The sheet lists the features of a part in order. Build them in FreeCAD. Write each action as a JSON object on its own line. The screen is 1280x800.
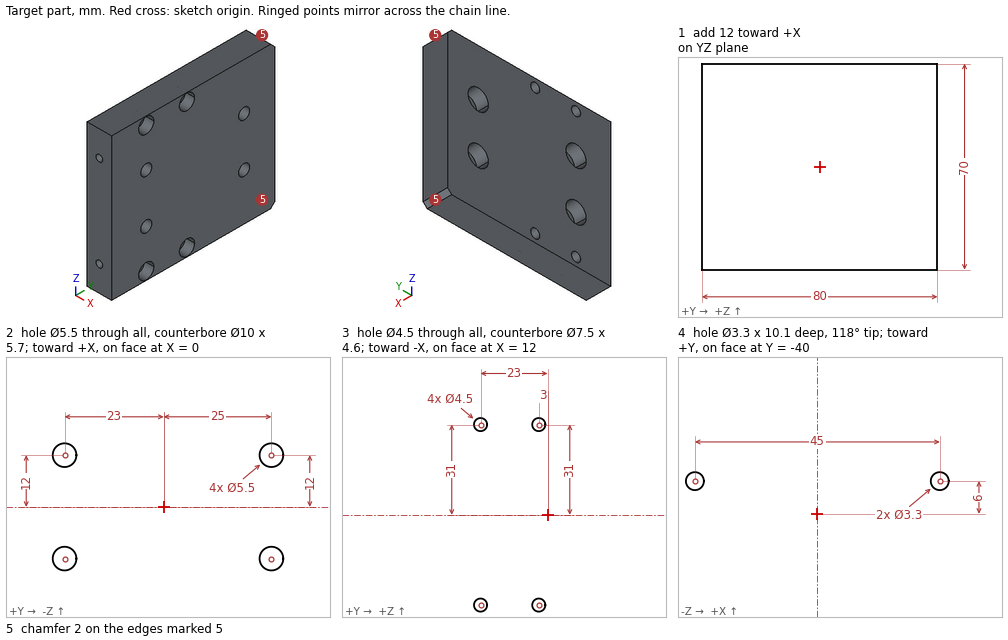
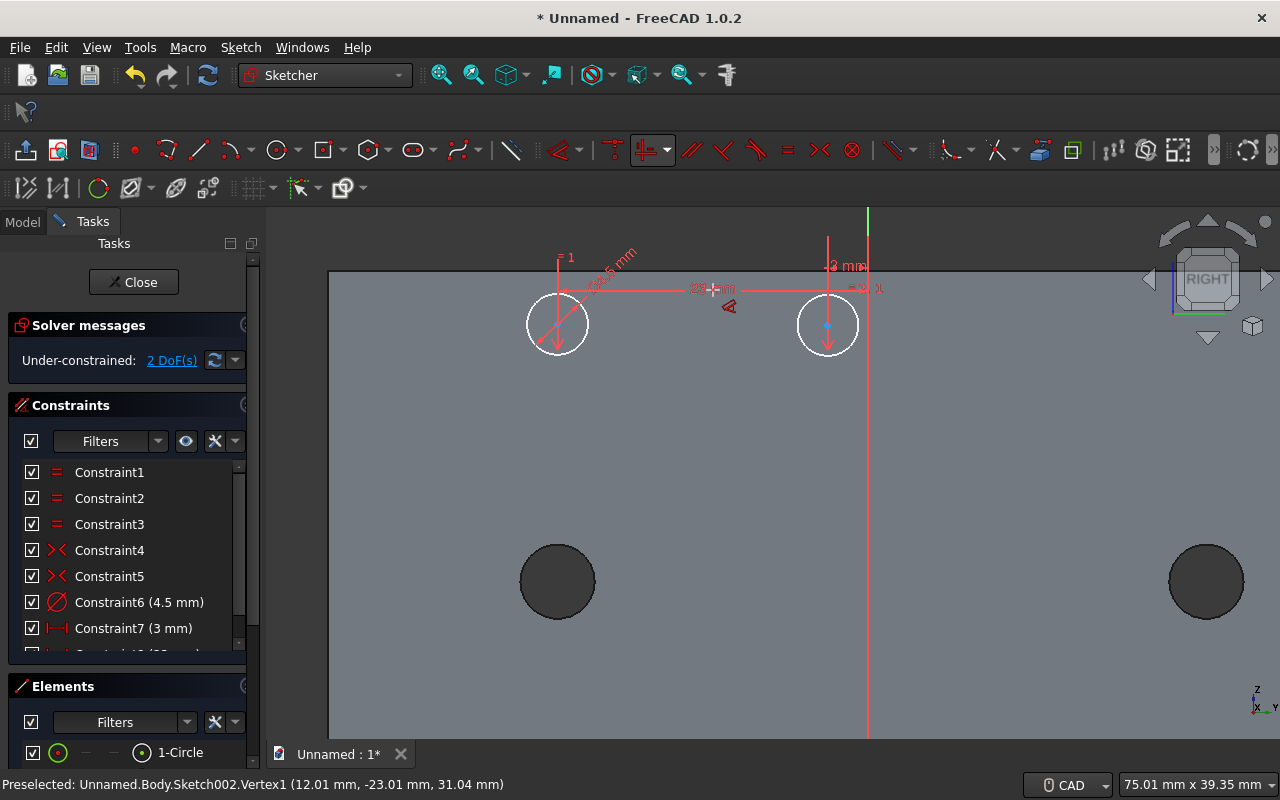
{"action": "left_click", "coordinate": [558, 324]}
{"action": "left_click", "coordinate": [902, 518]}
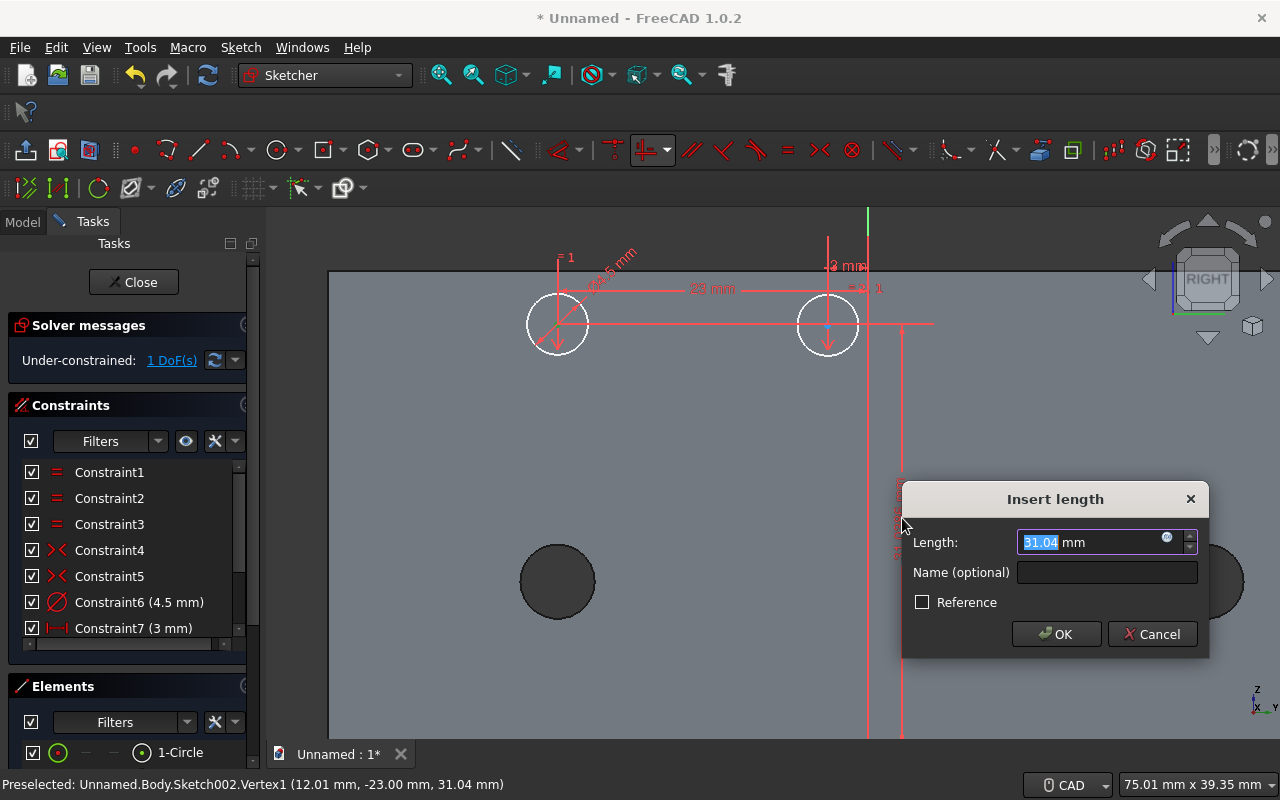
{"action": "type", "text": "31"}
{"action": "key", "text": "Return"}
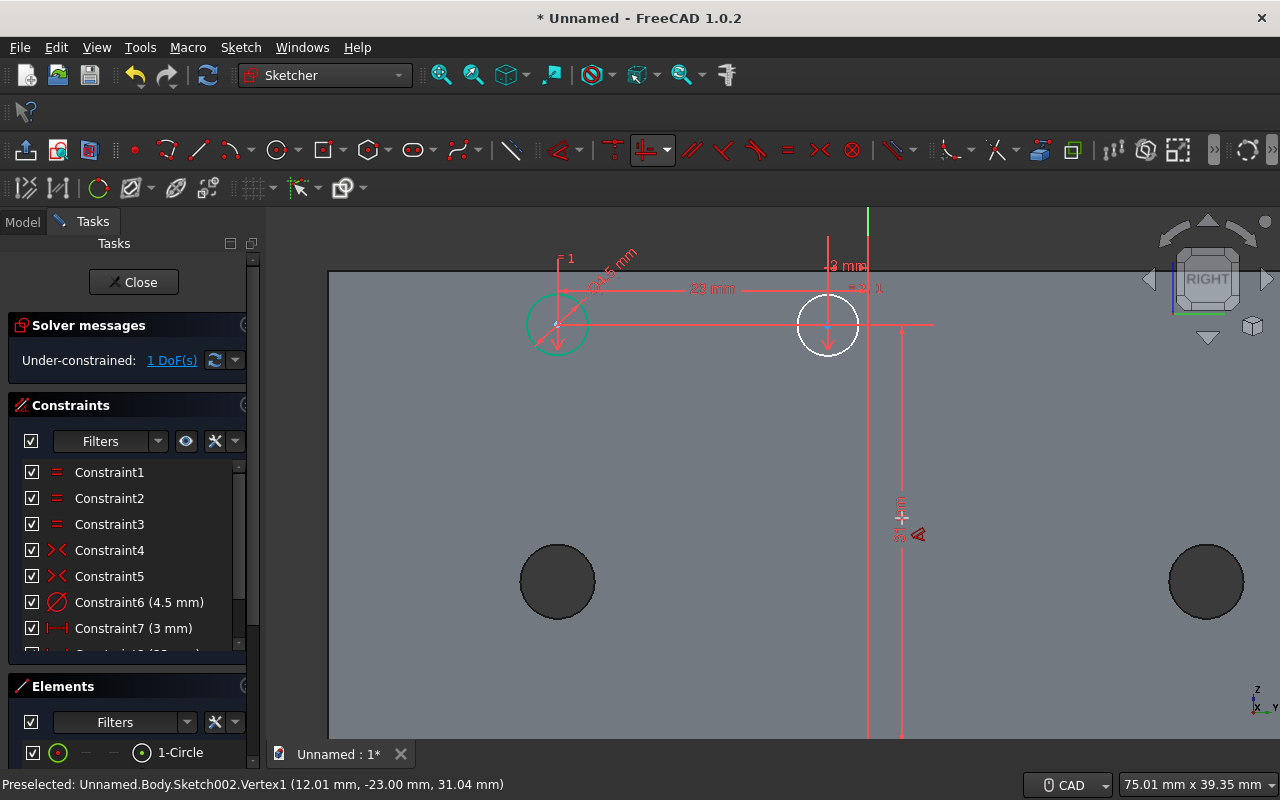
{"action": "left_click", "coordinate": [828, 325]}
{"action": "left_click", "coordinate": [902, 430]}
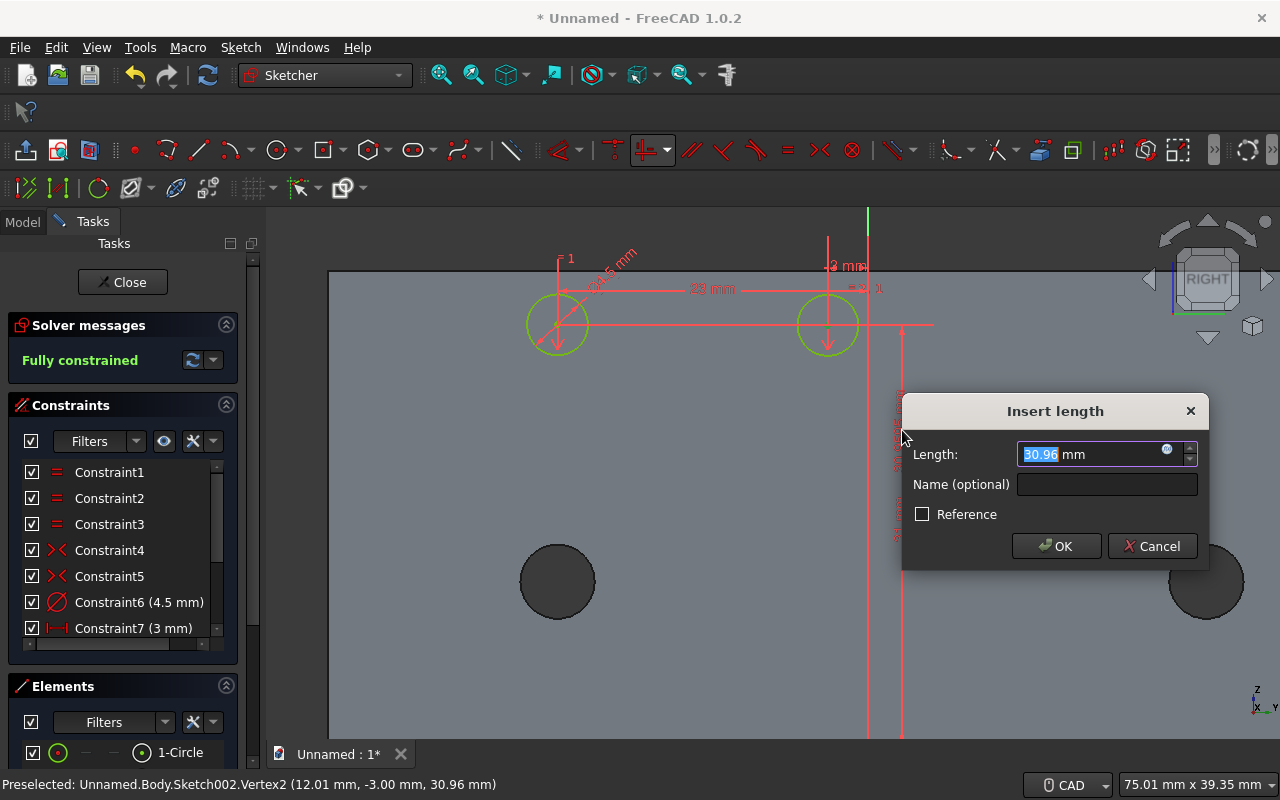
{"action": "type", "text": "31"}
{"action": "key", "text": "Return"}
{"action": "key", "text": "Escape"}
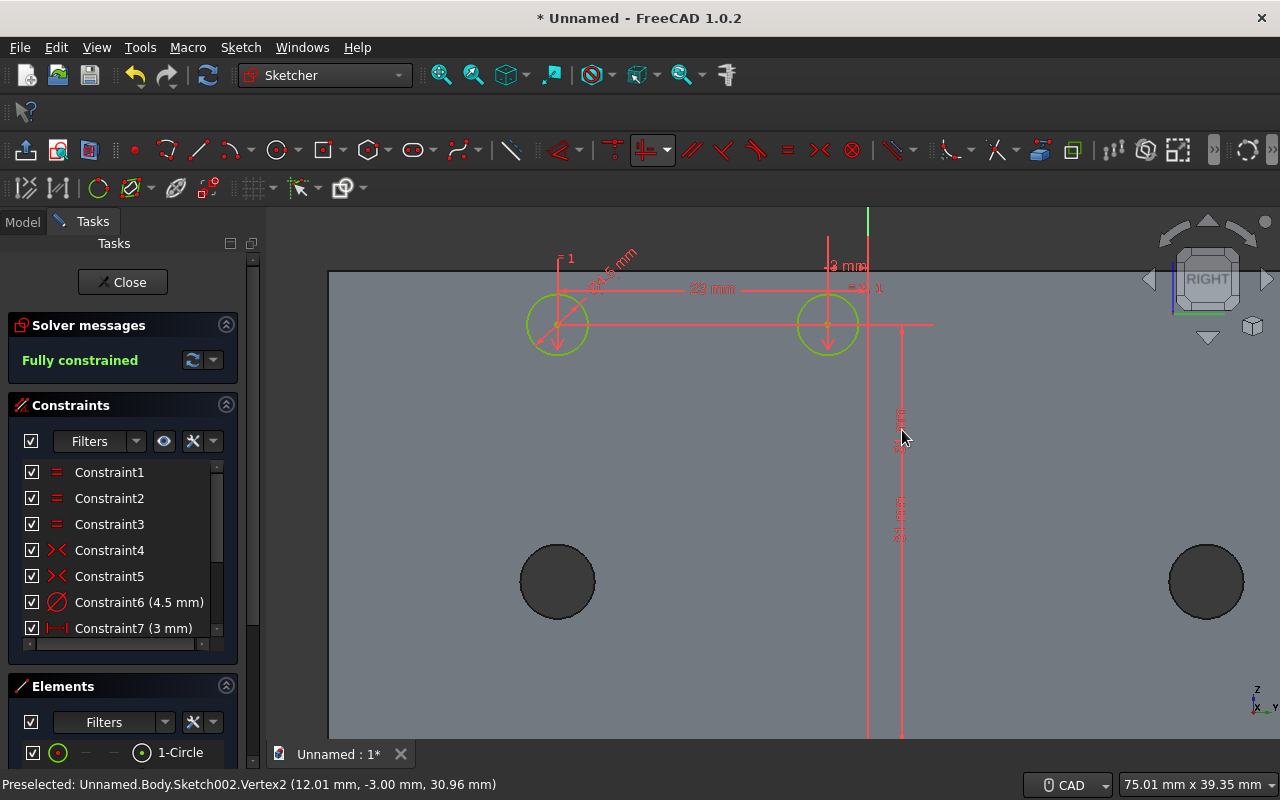
{"action": "left_click", "coordinate": [123, 282]}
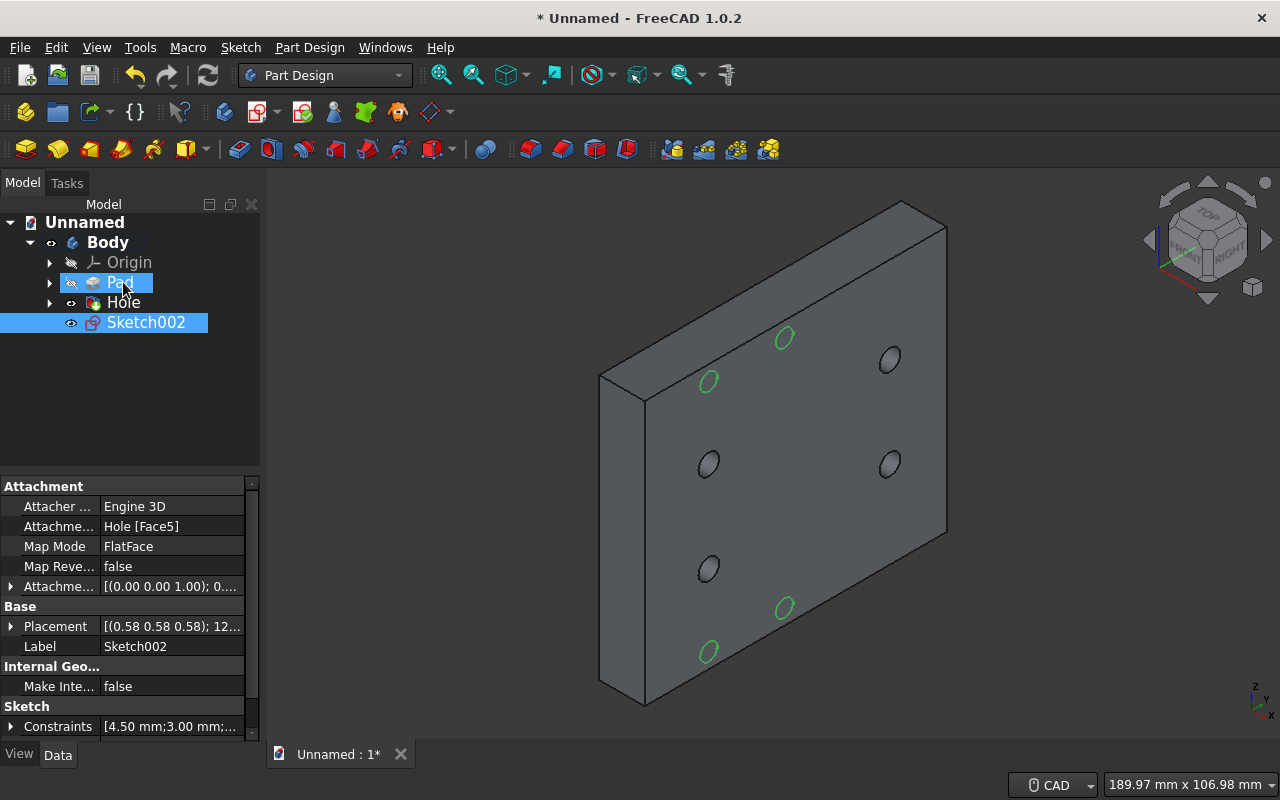
{"action": "left_click", "coordinate": [272, 150]}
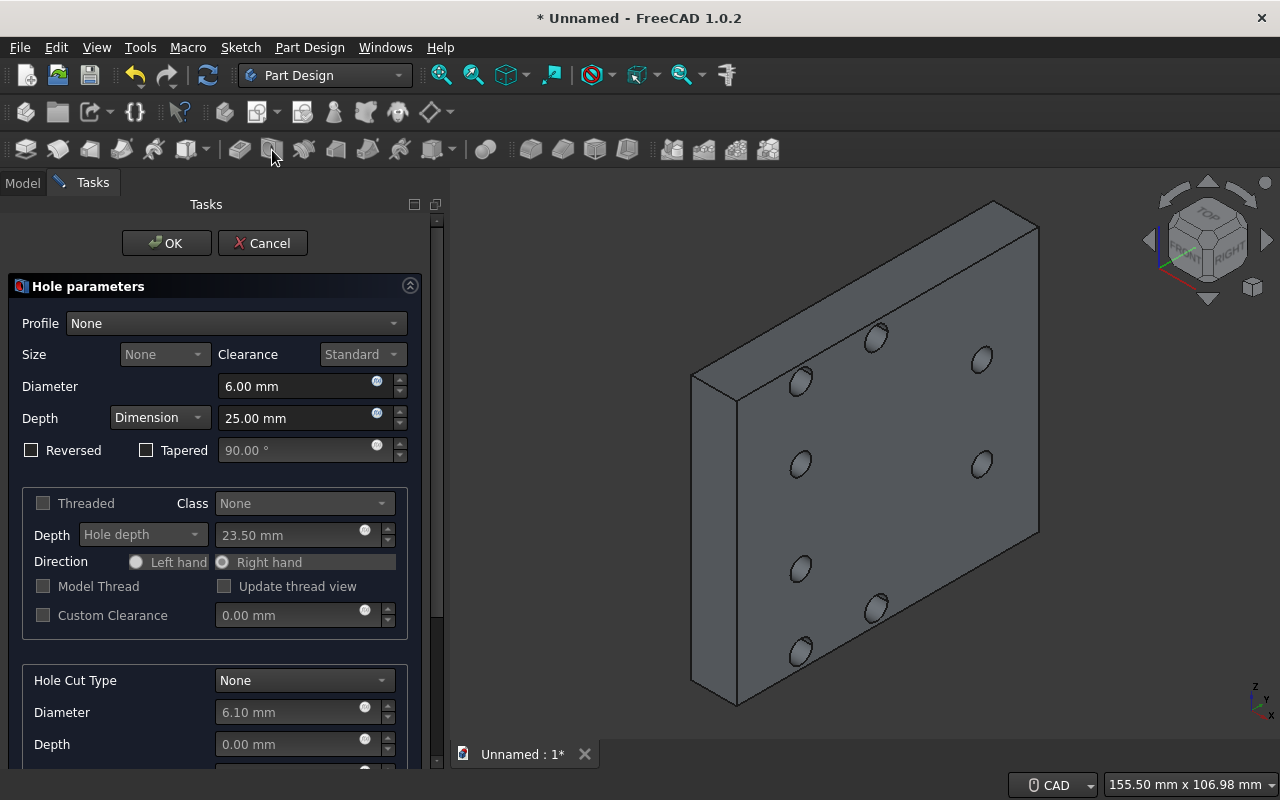
{"action": "triple_click", "coordinate": [305, 386]}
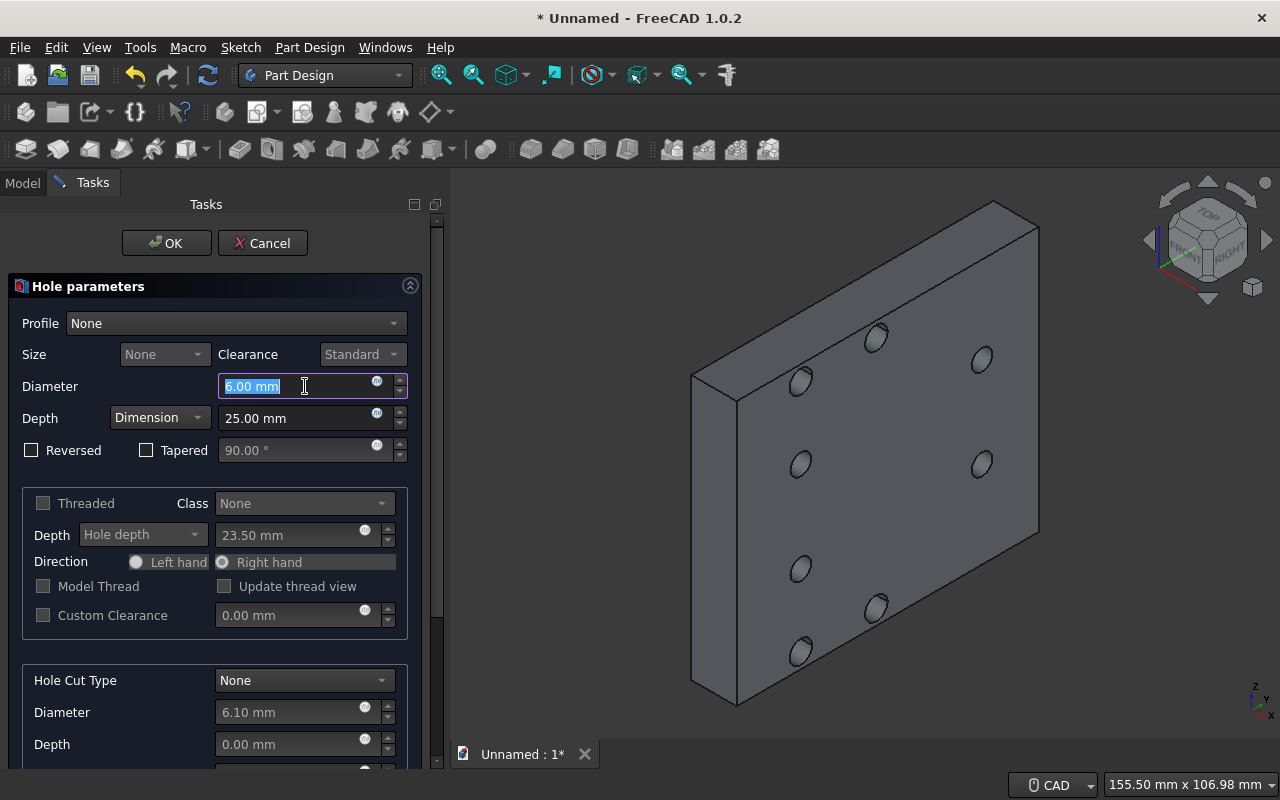
{"action": "type", "text": "4.5"}
{"action": "key", "text": "Tab"}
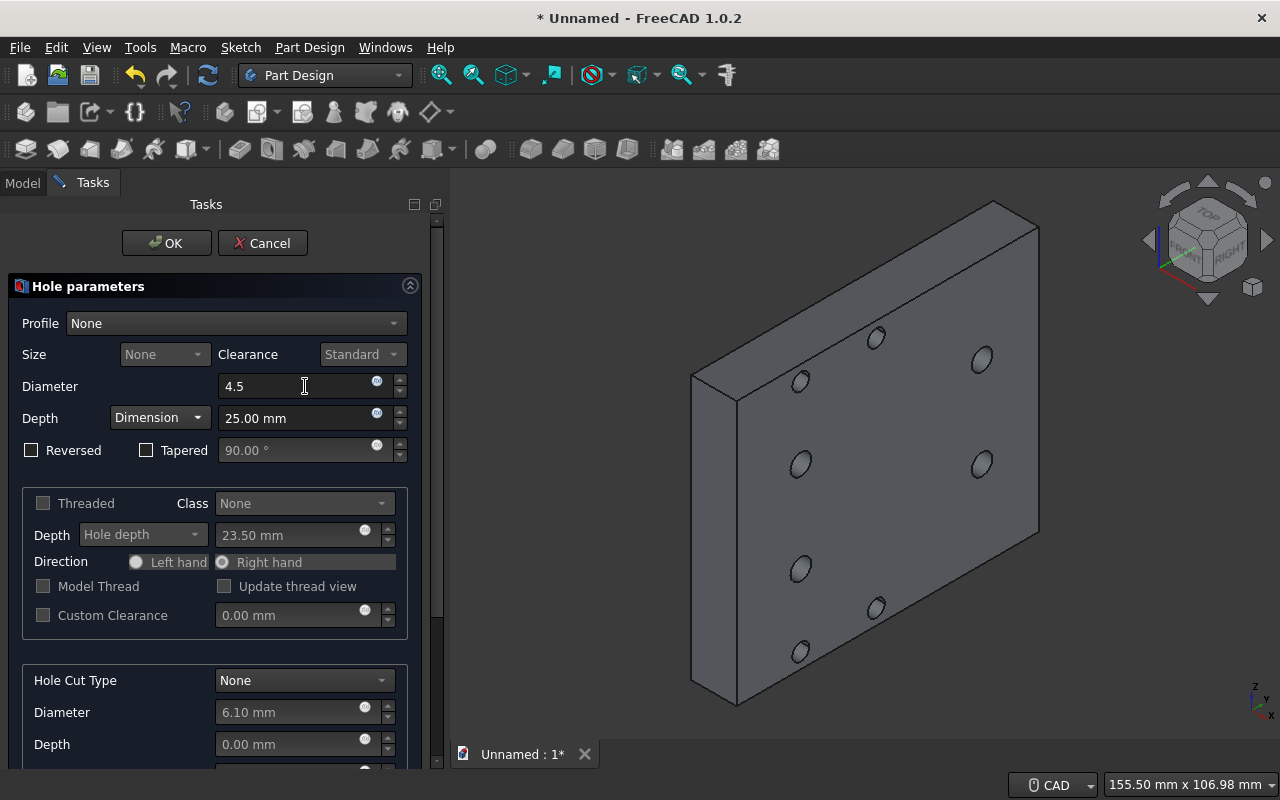
{"action": "left_click", "coordinate": [161, 418]}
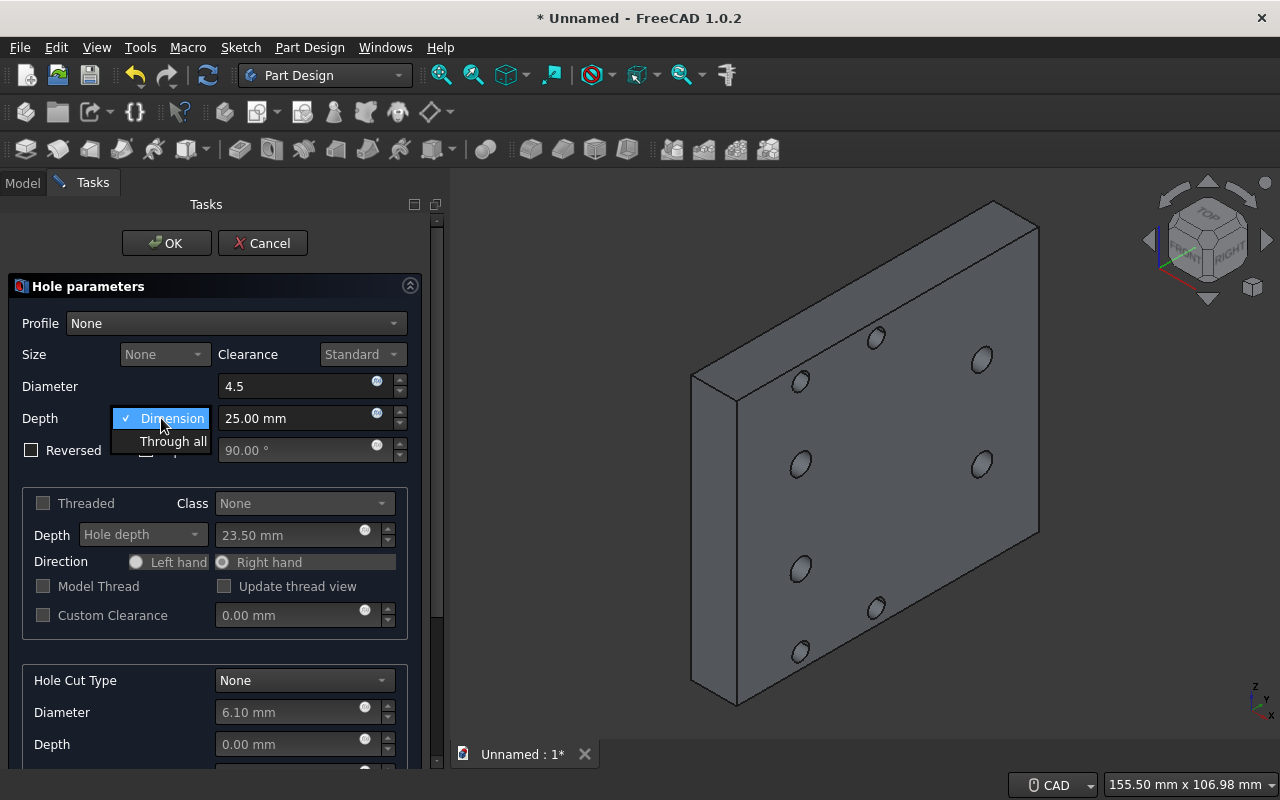
{"action": "left_click", "coordinate": [160, 442]}